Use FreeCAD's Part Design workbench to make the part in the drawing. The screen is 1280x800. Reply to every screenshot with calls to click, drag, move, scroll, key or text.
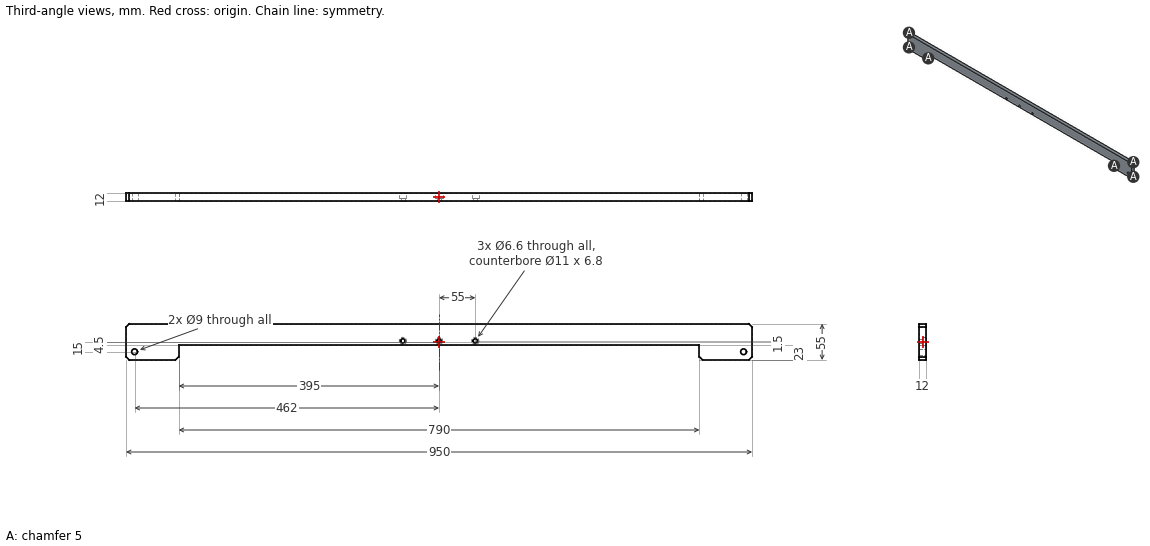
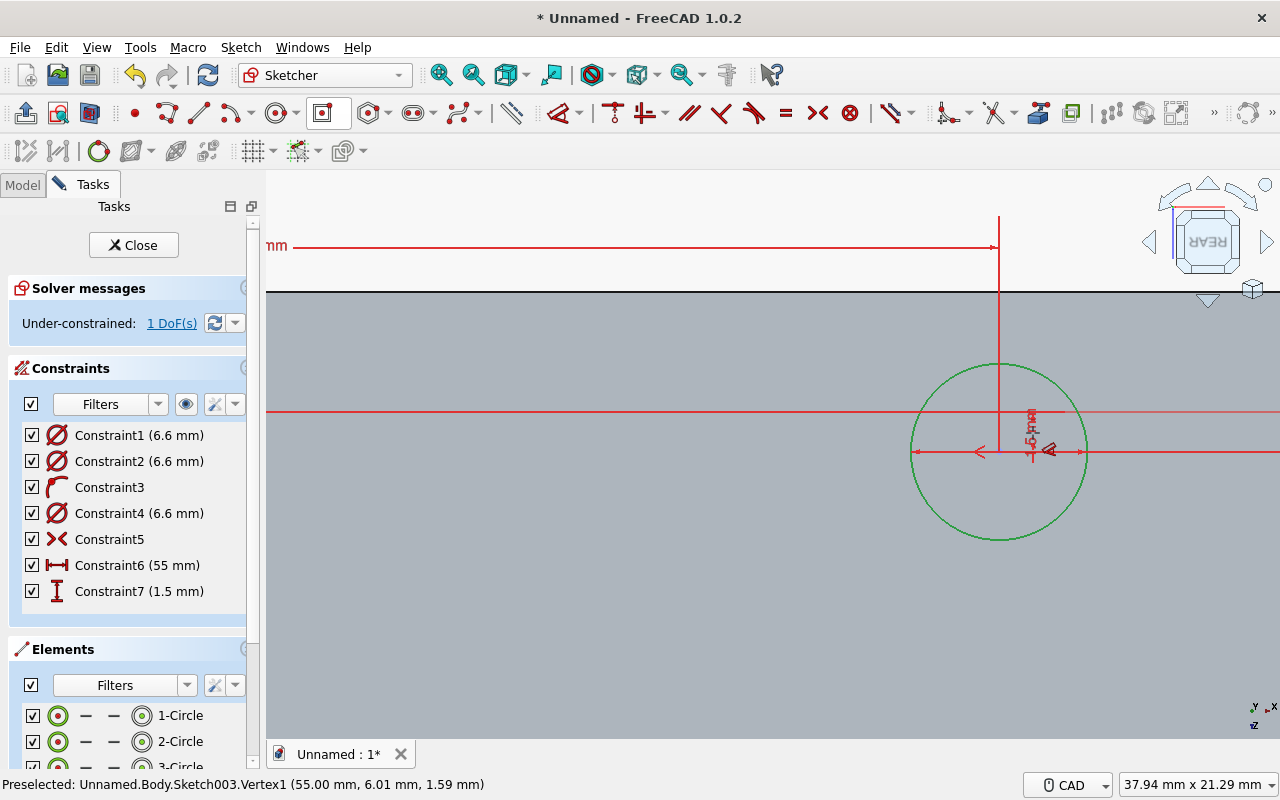
scroll(1002, 455, down, 8)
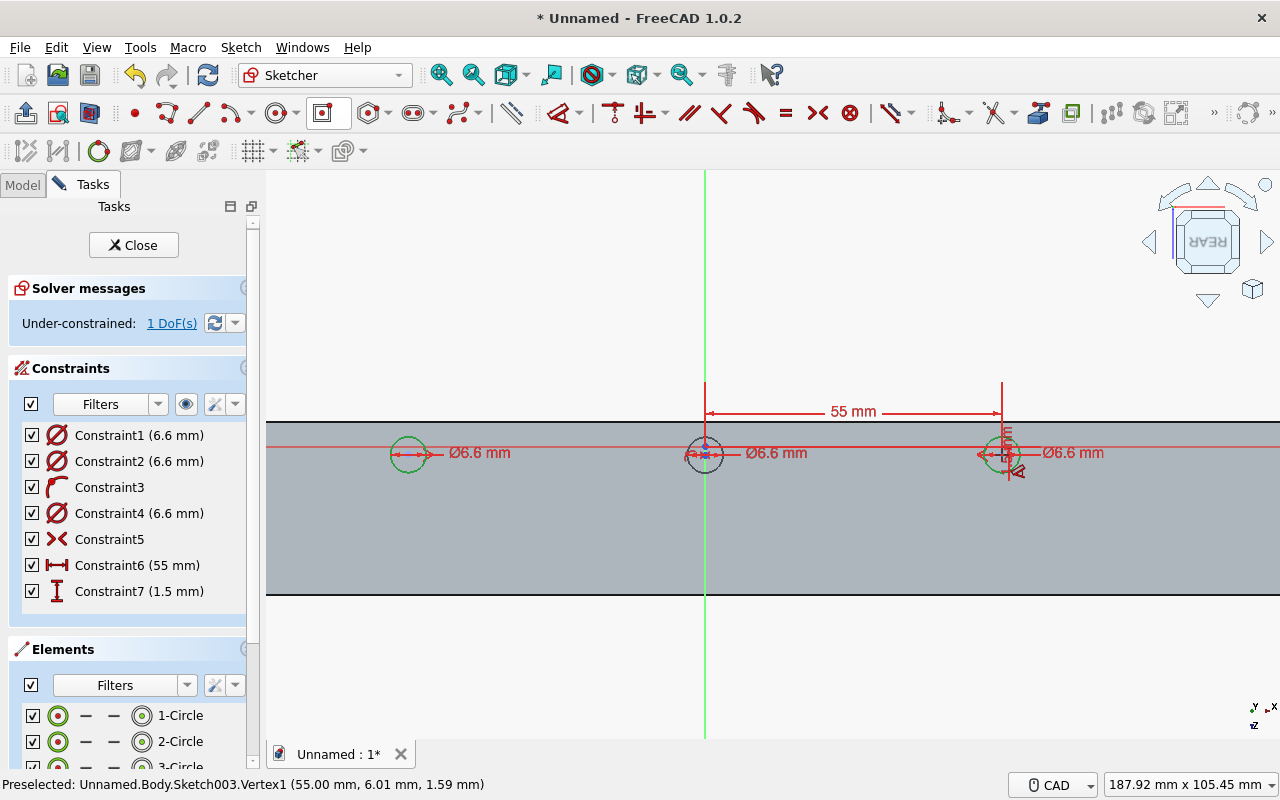
scroll(705, 455, up, 8)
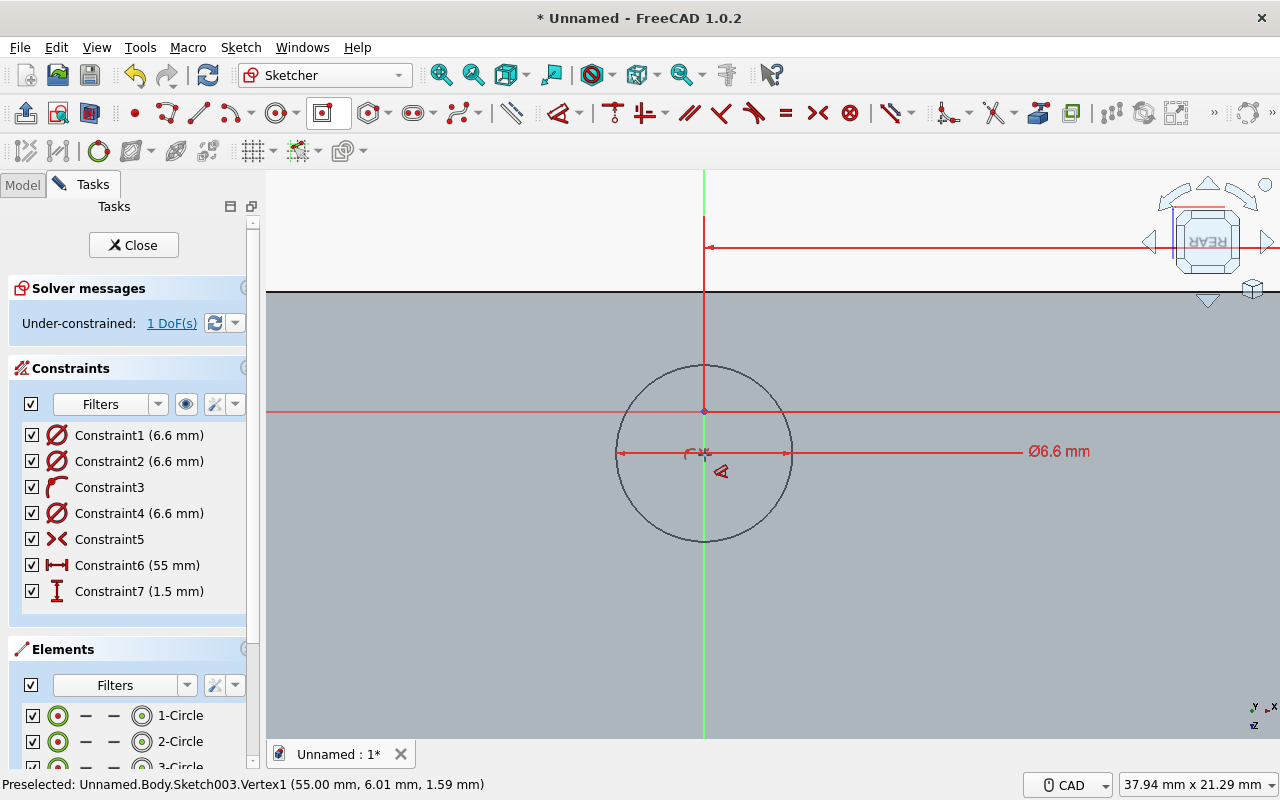
click(704, 453)
click(738, 433)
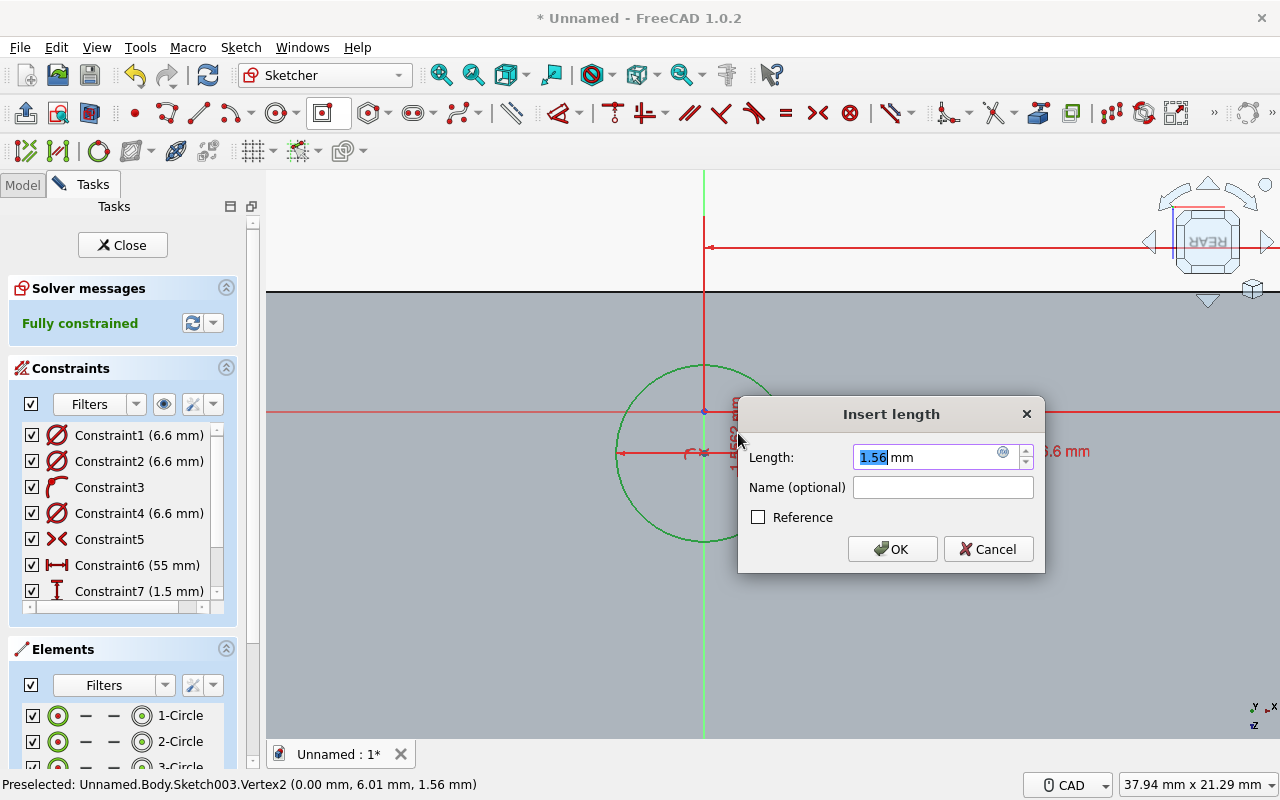
text(1.5)
key(Return)
key(Escape)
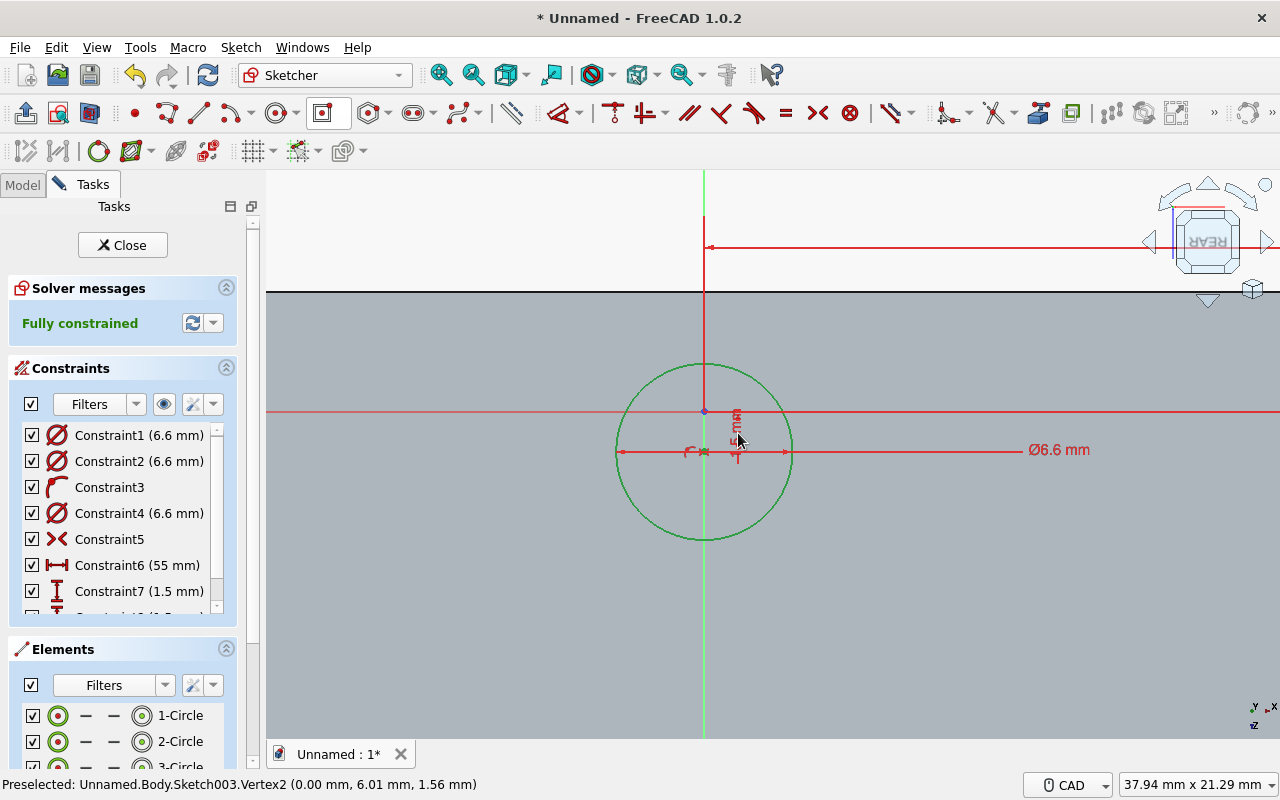
click(123, 245)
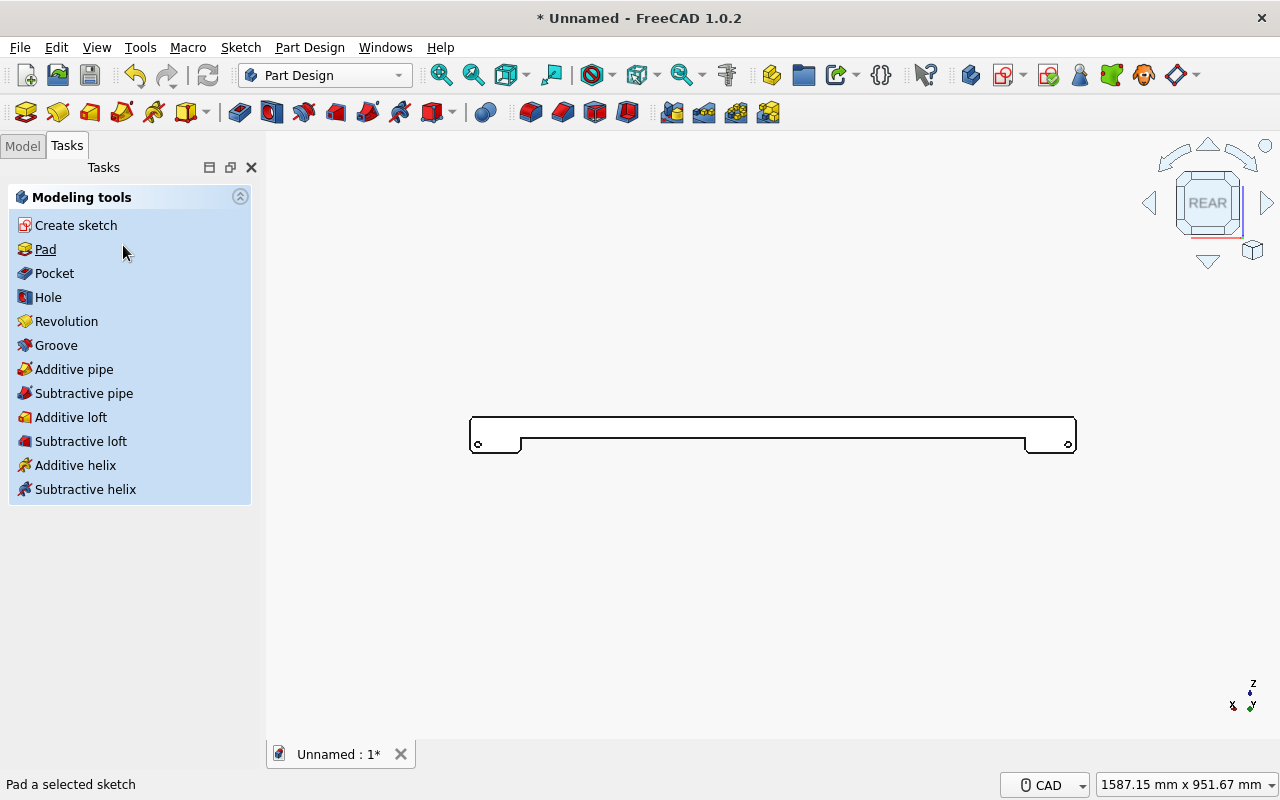
click(272, 112)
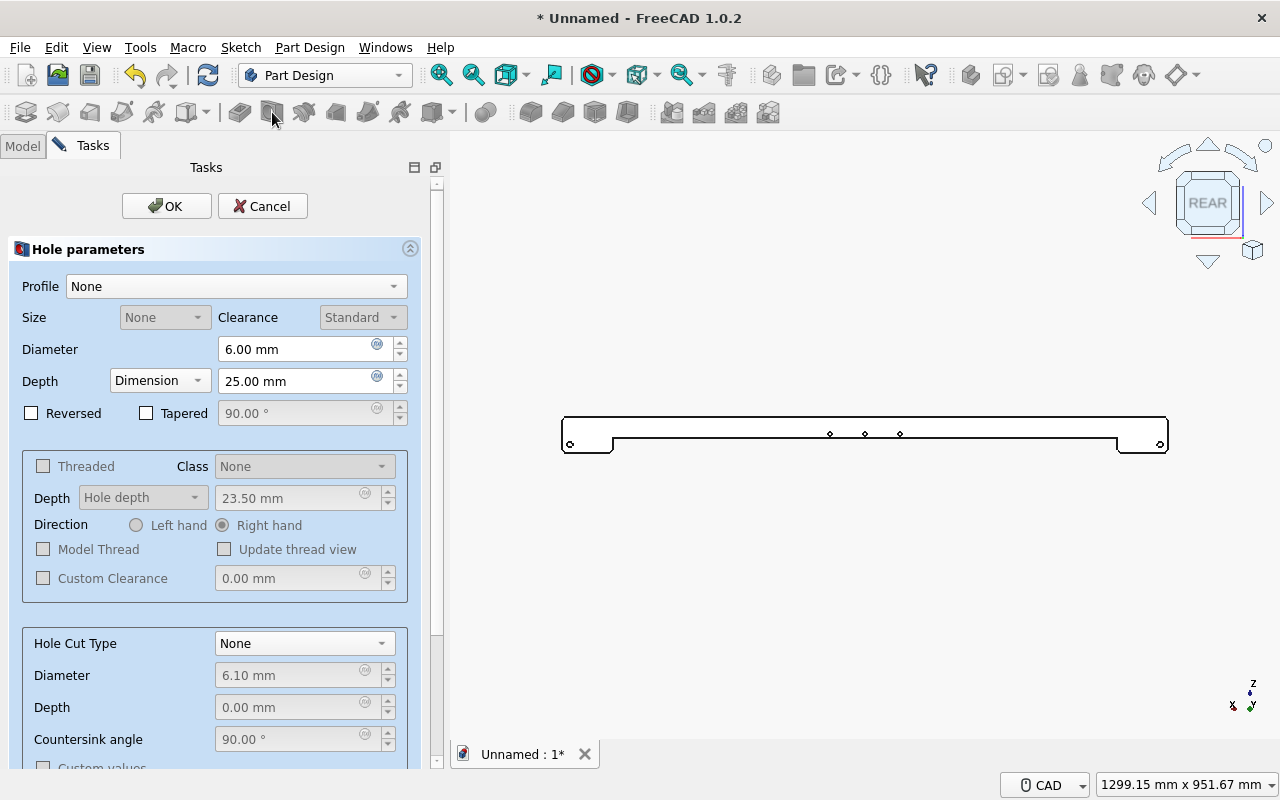
triple_click(305, 349)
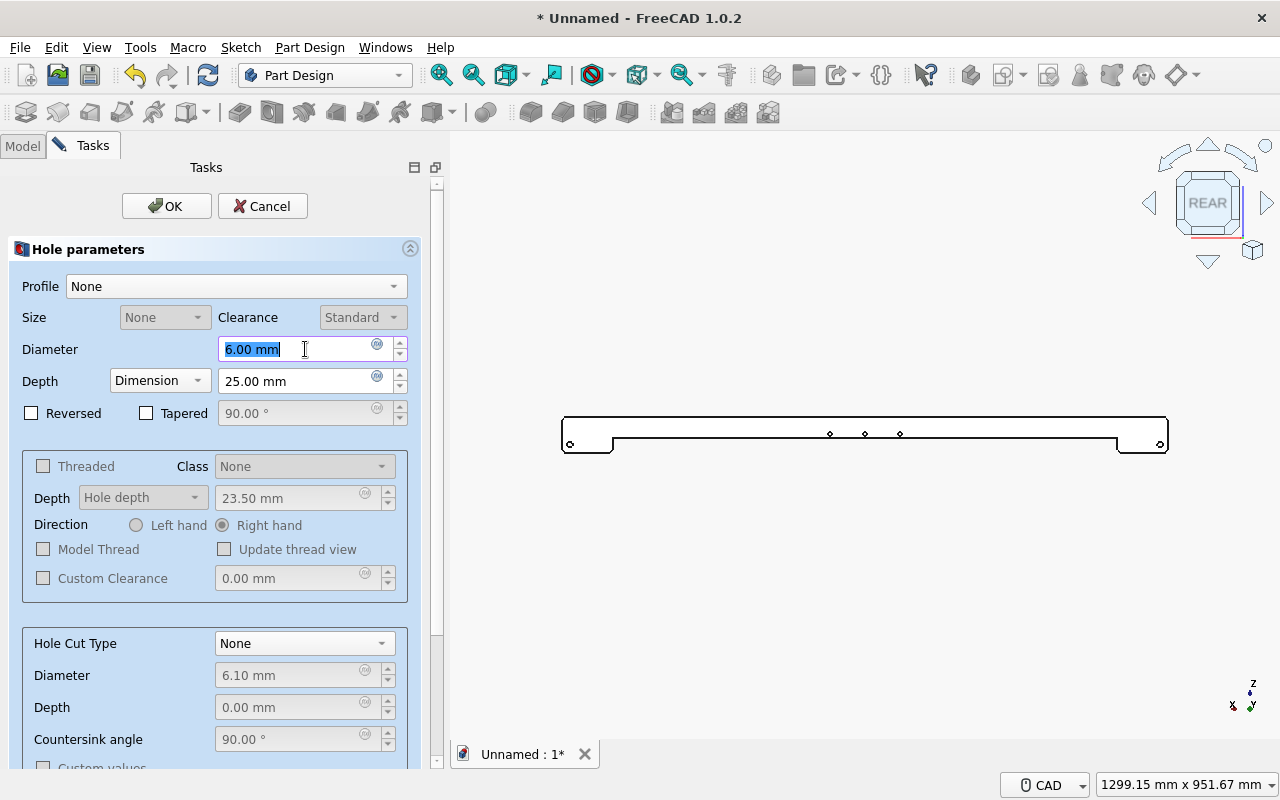
text(6.6)
key(Tab)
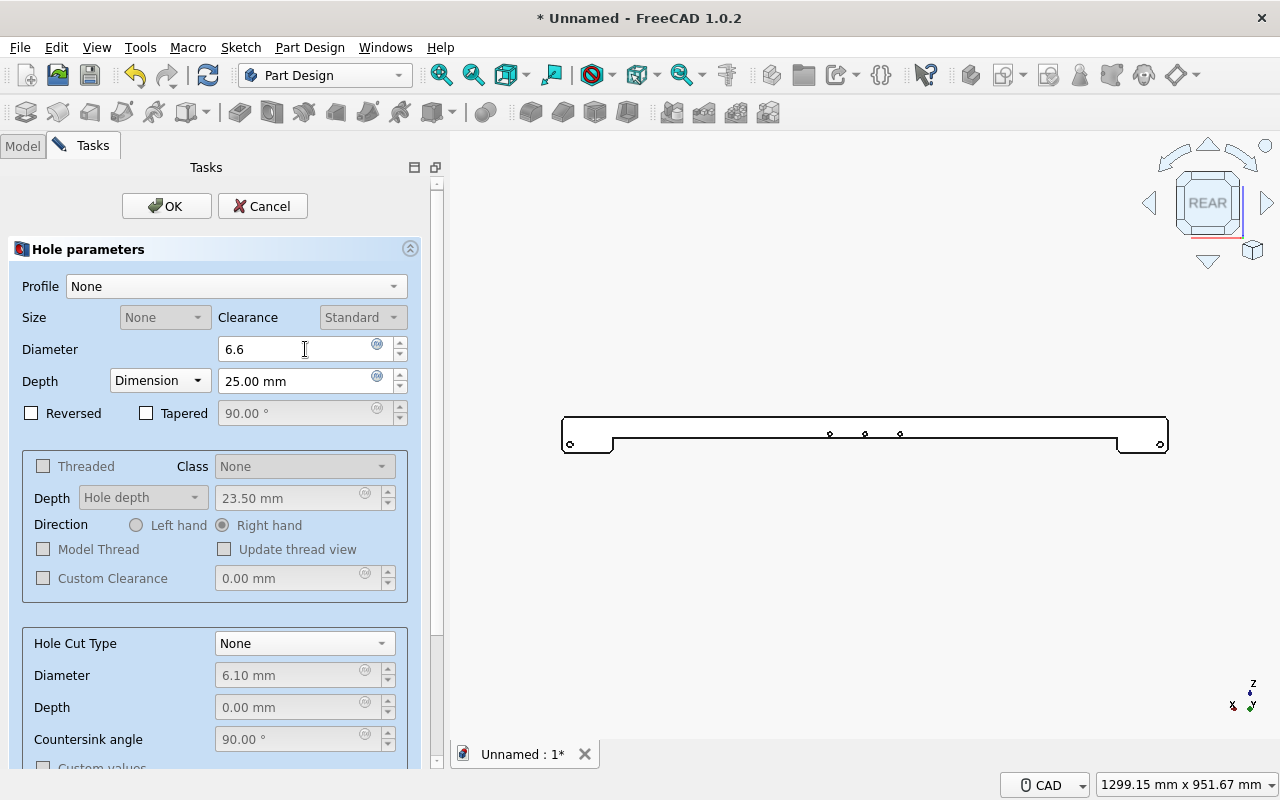
click(161, 380)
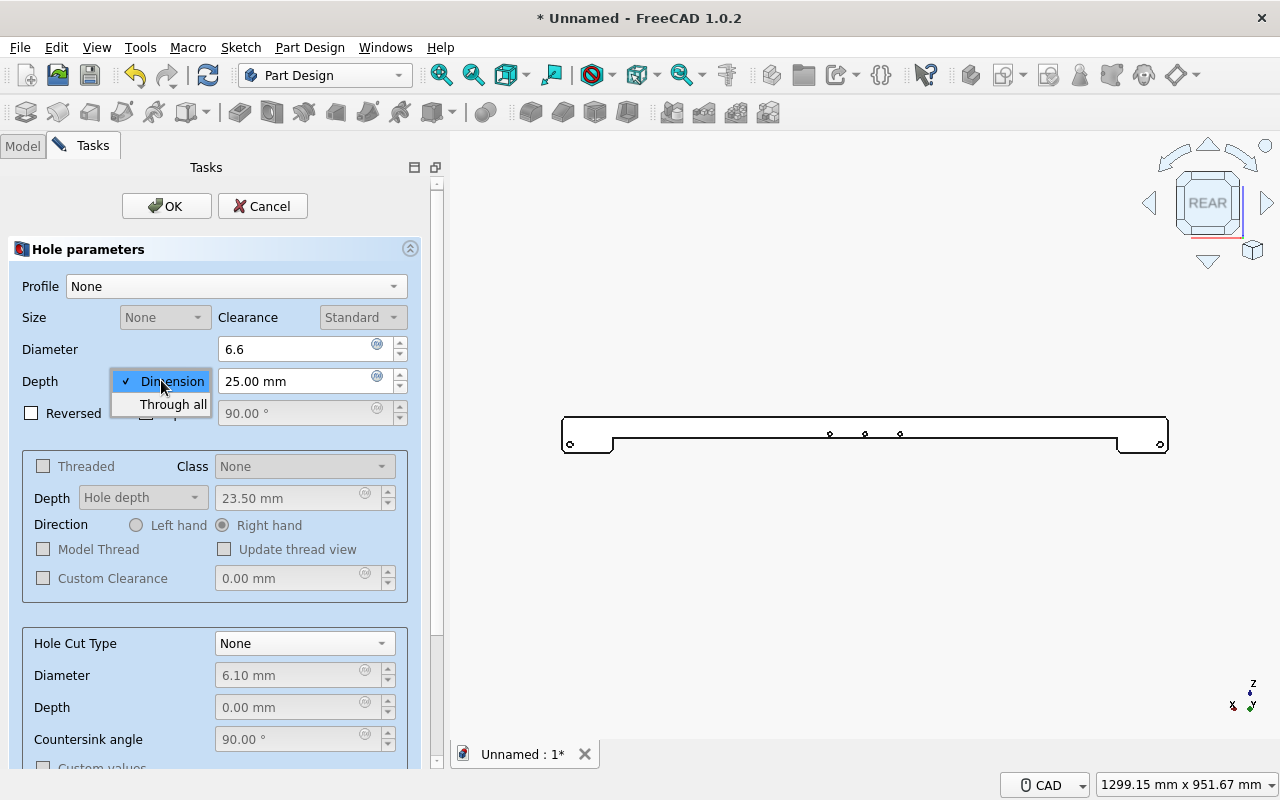
click(160, 404)